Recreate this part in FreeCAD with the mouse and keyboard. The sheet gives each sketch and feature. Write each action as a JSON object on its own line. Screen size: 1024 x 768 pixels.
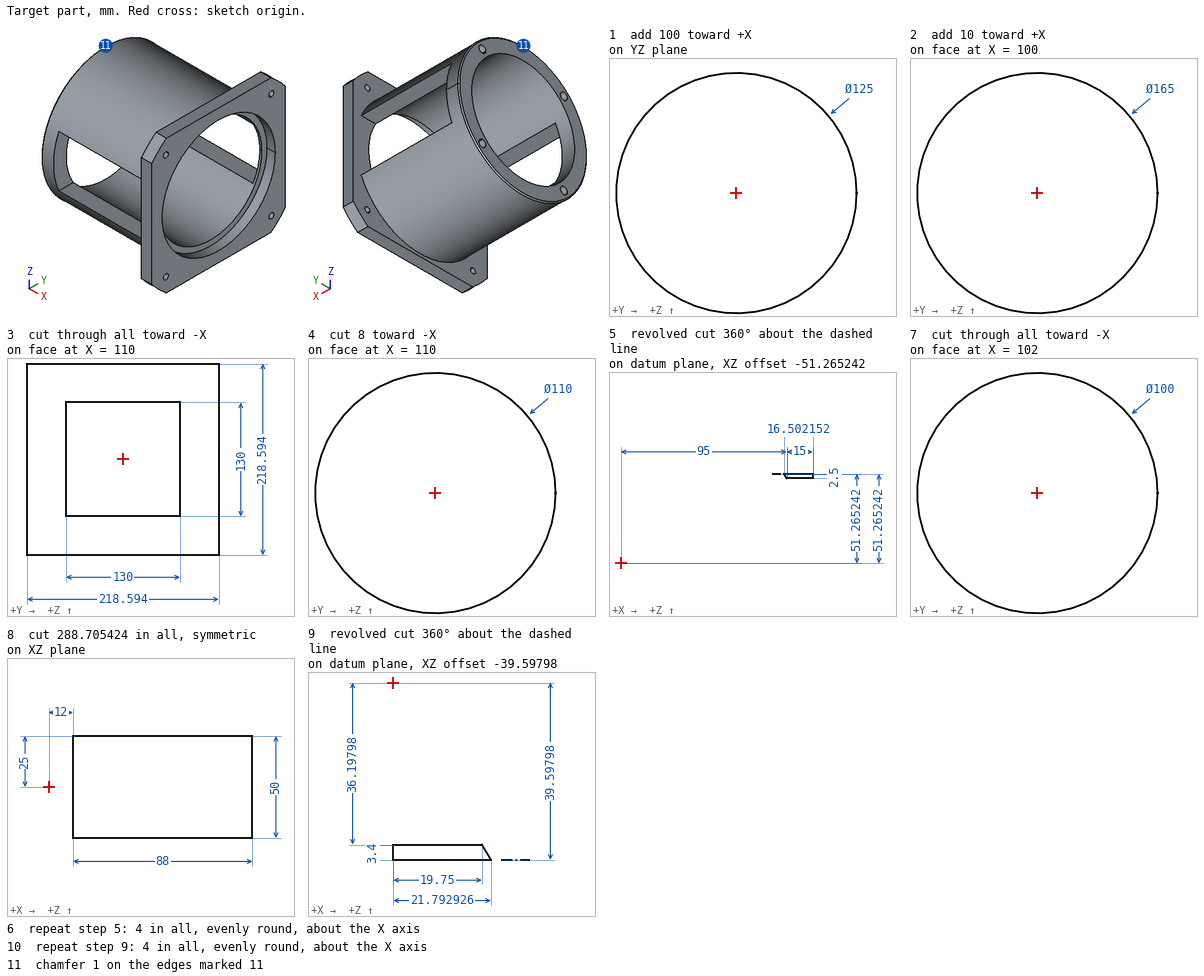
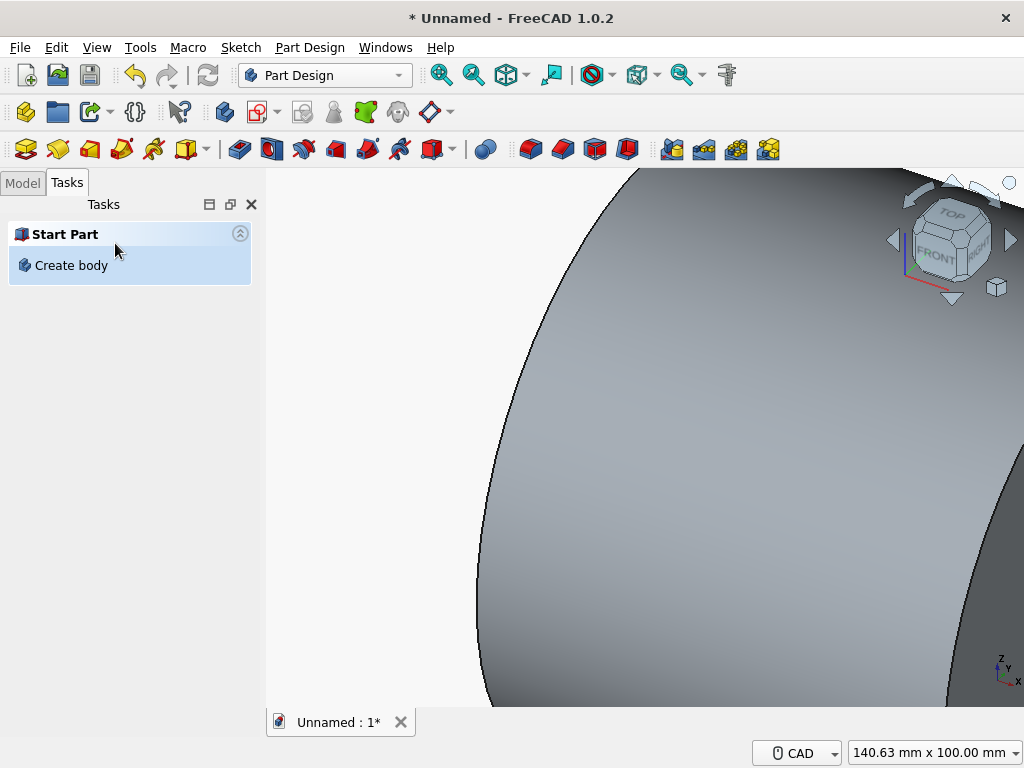
{"action": "left_click", "coordinate": [442, 76]}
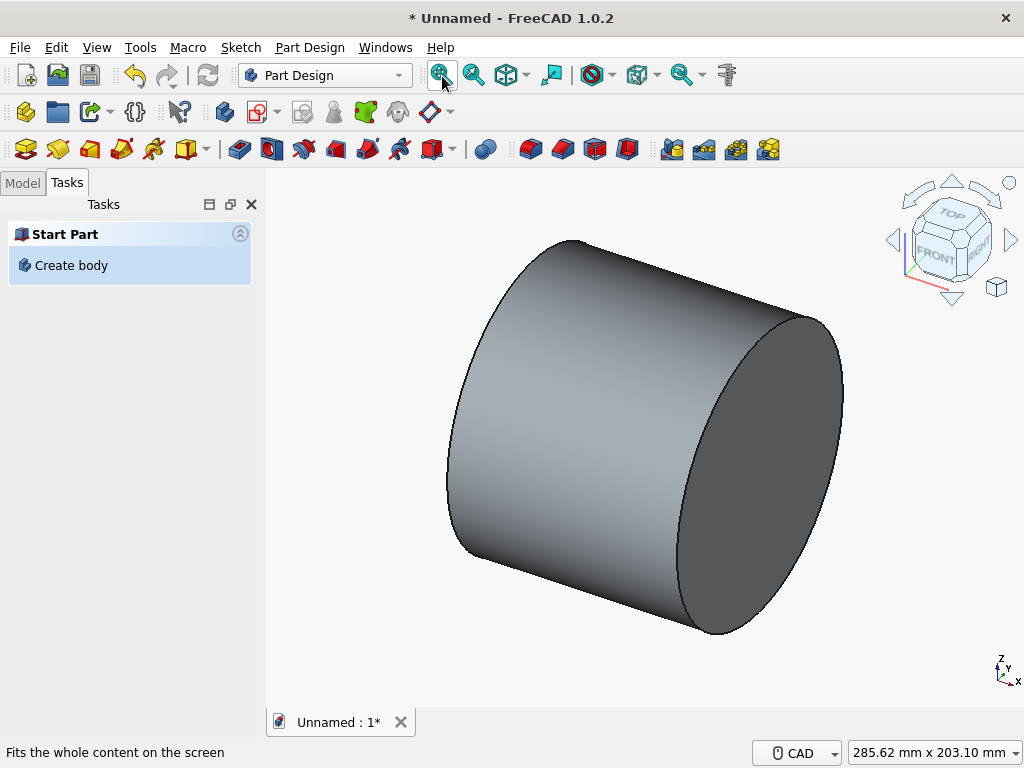
{"action": "left_click", "coordinate": [760, 475]}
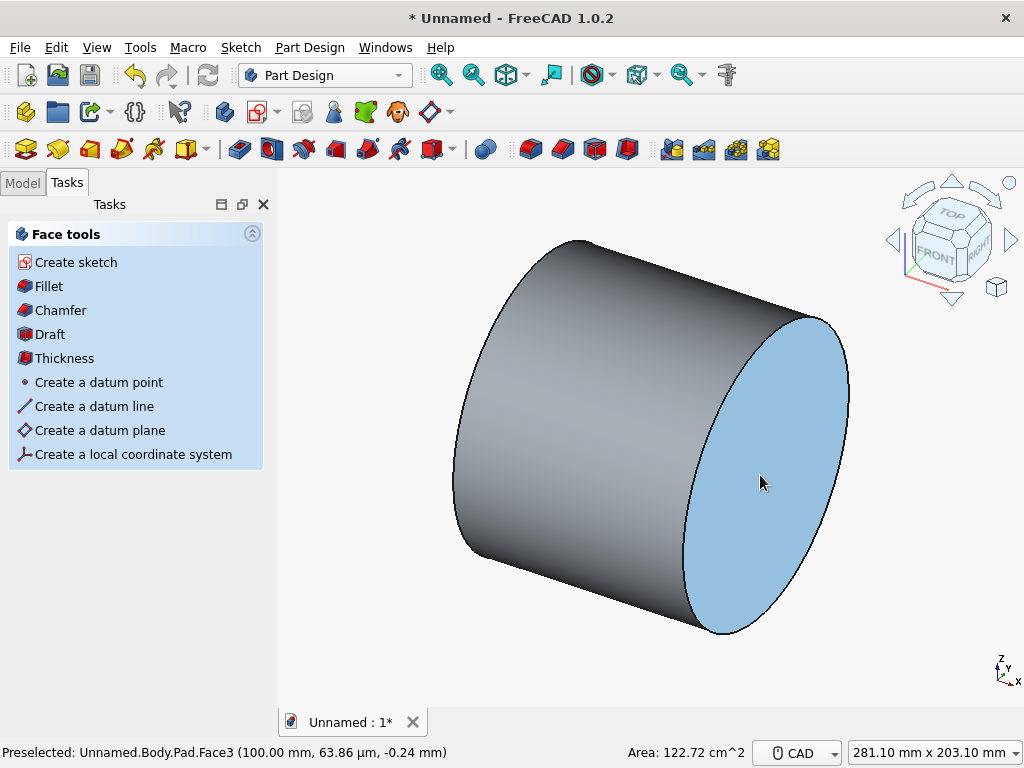
{"action": "left_click", "coordinate": [258, 112]}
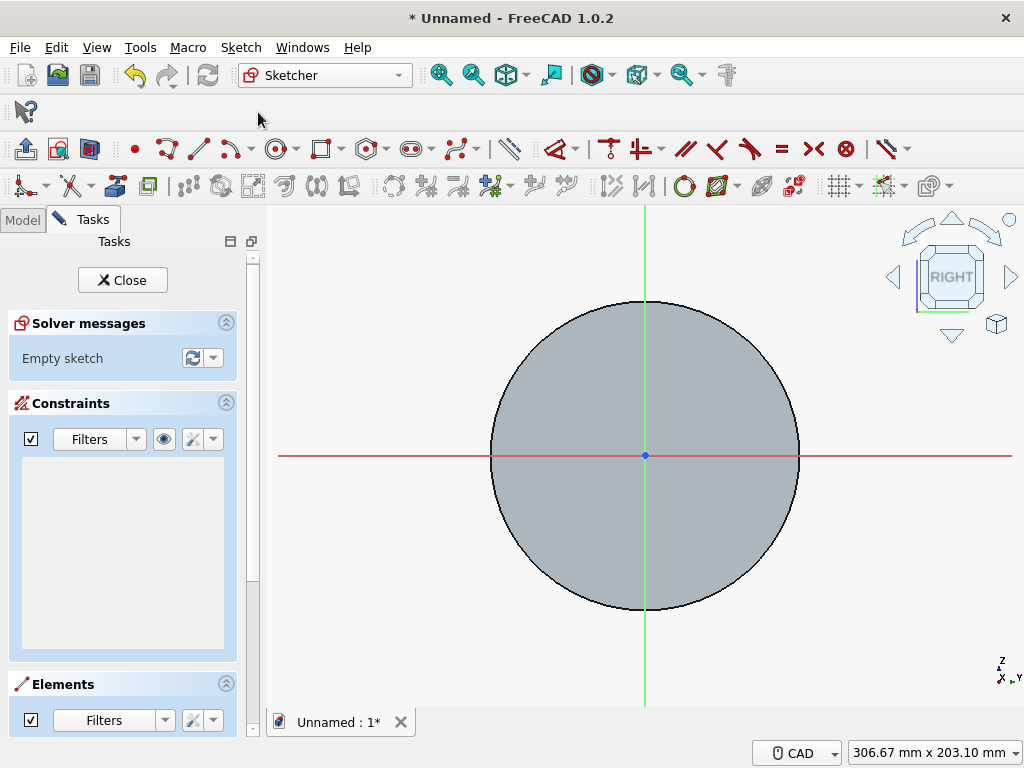
{"action": "scroll", "coordinate": [294, 456], "scroll_direction": "down", "scroll_amount": 1}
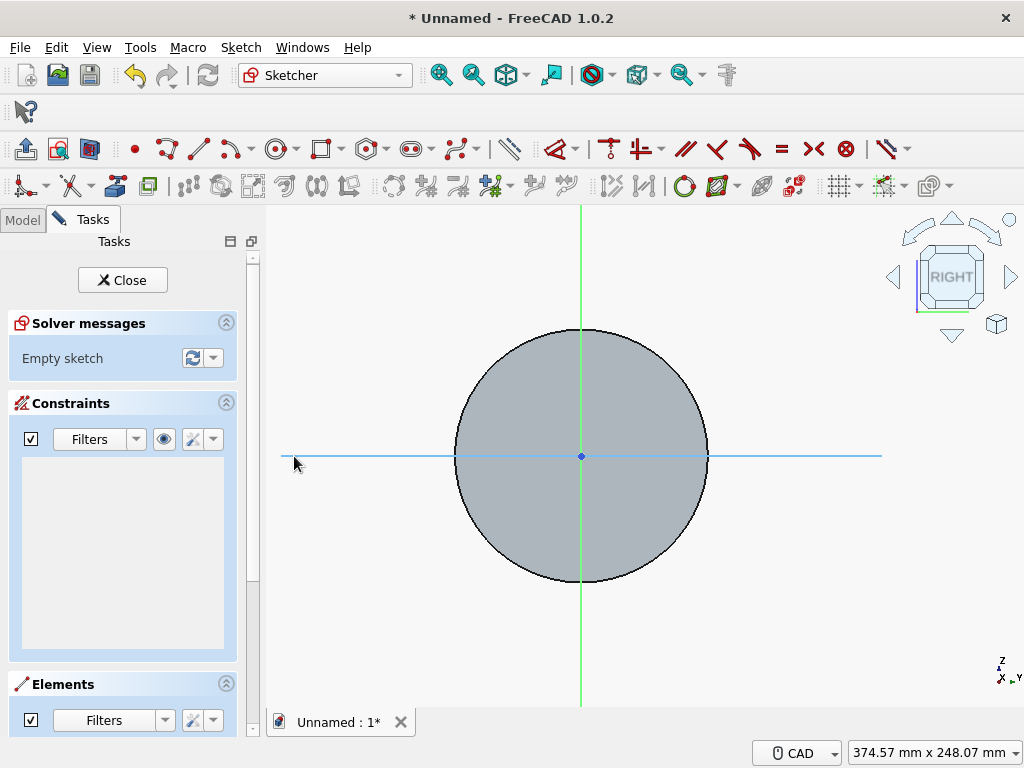
{"action": "left_click", "coordinate": [276, 150]}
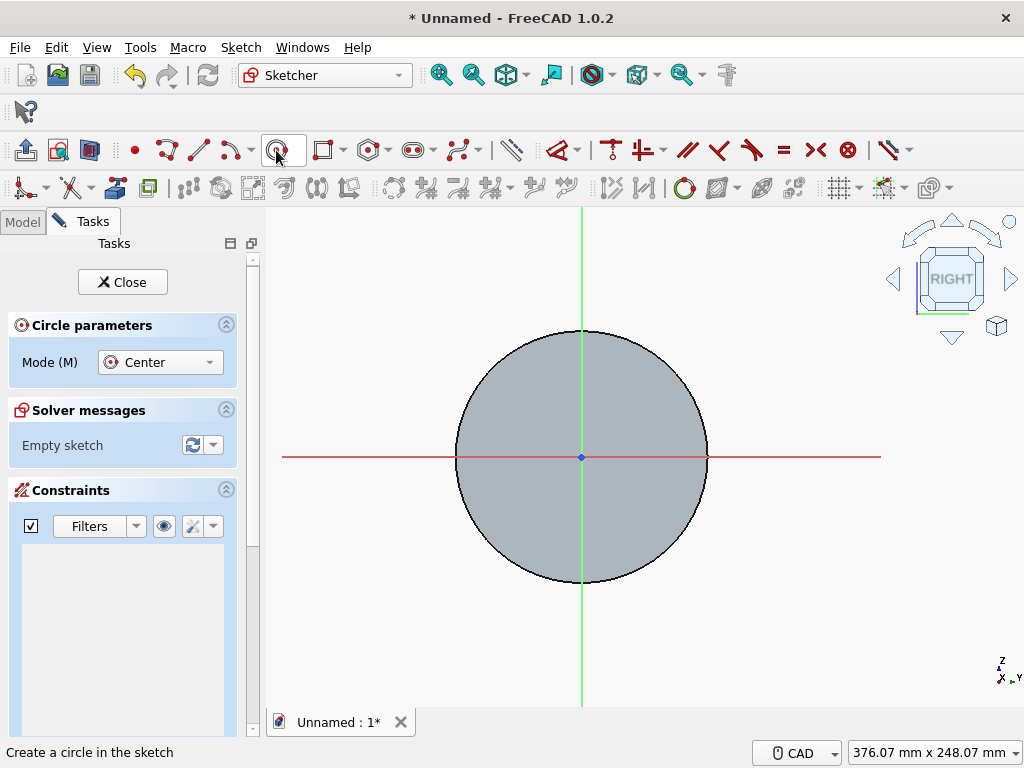
{"action": "left_click", "coordinate": [582, 457]}
{"action": "mouse_move", "coordinate": [699, 340]}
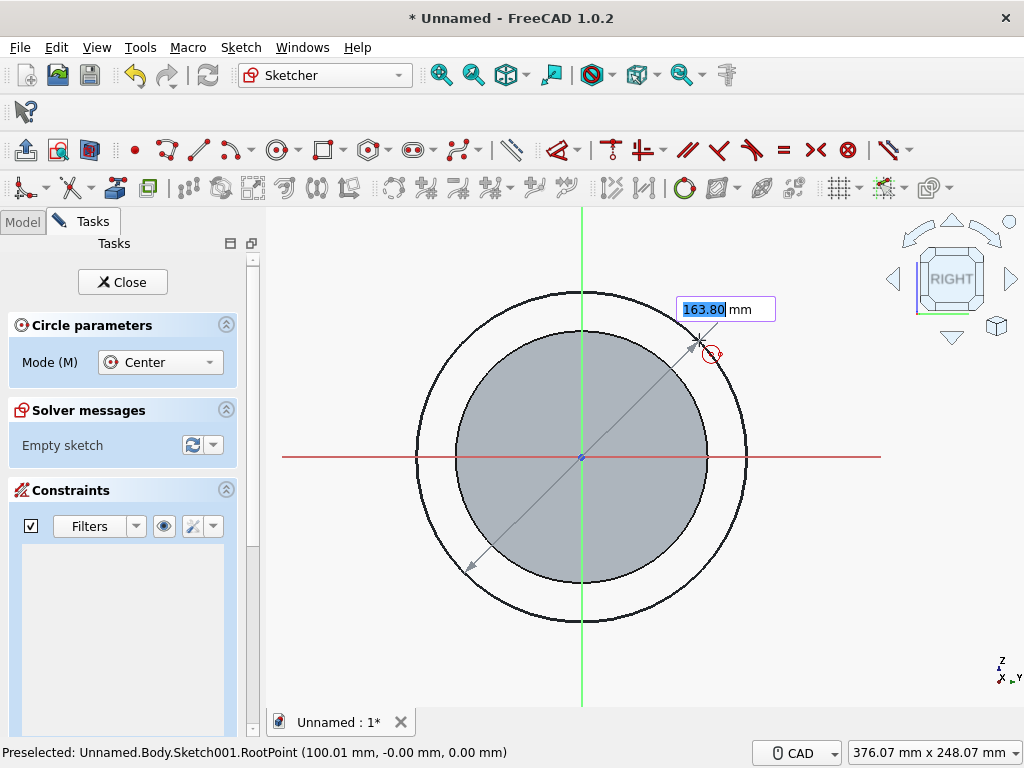
{"action": "type", "text": "165"}
{"action": "key", "text": "Return"}
{"action": "key", "text": "Escape"}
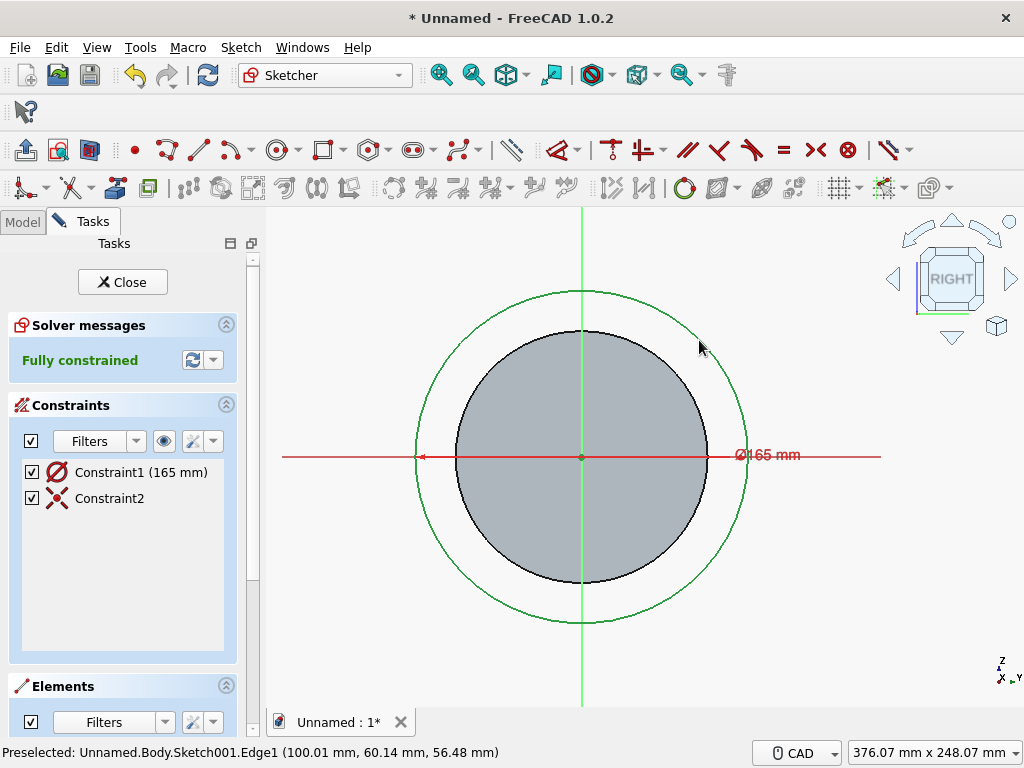
{"action": "left_click", "coordinate": [123, 282]}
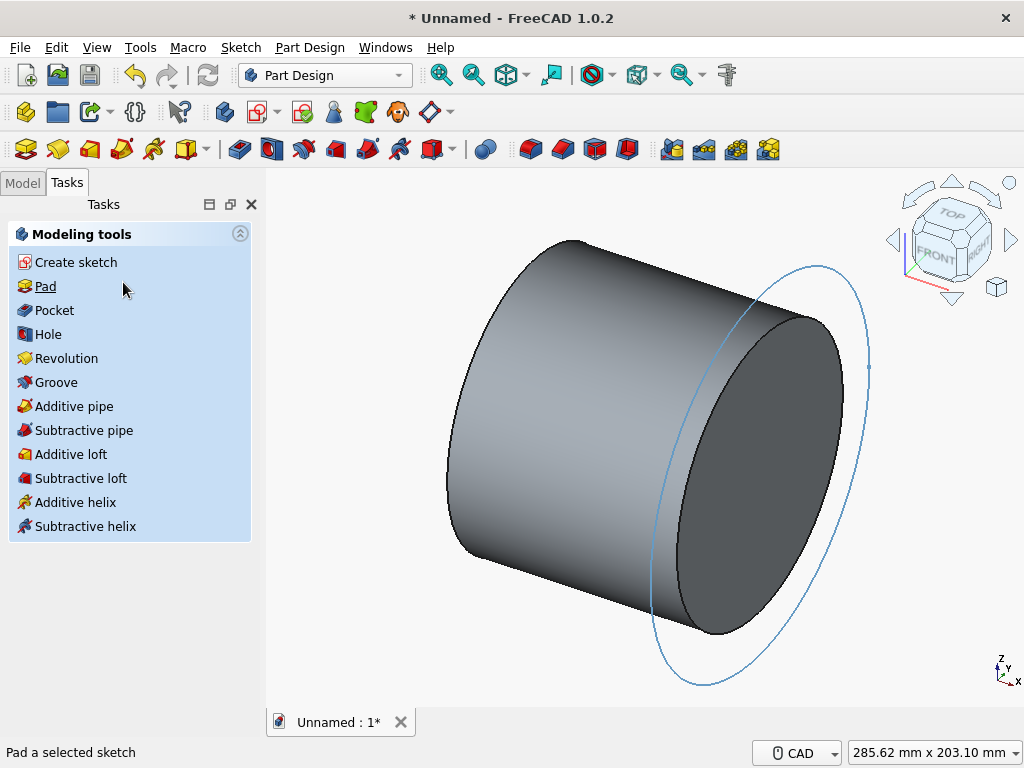
{"action": "left_click", "coordinate": [26, 150]}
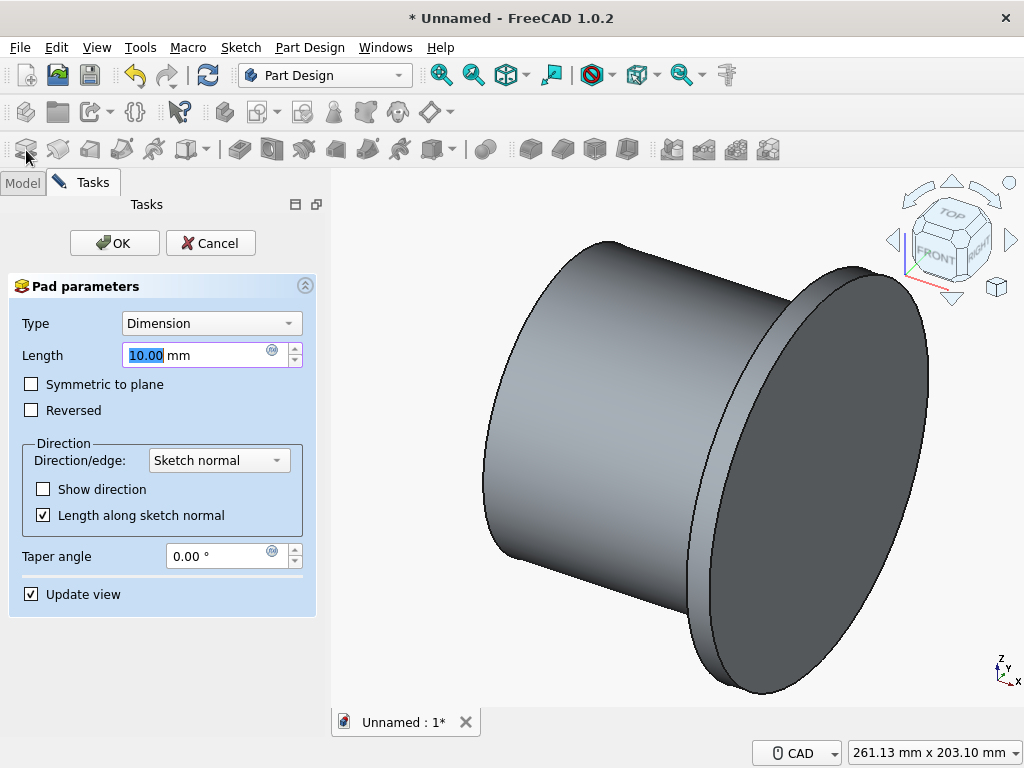
{"action": "type", "text": "10"}
{"action": "key", "text": "Tab"}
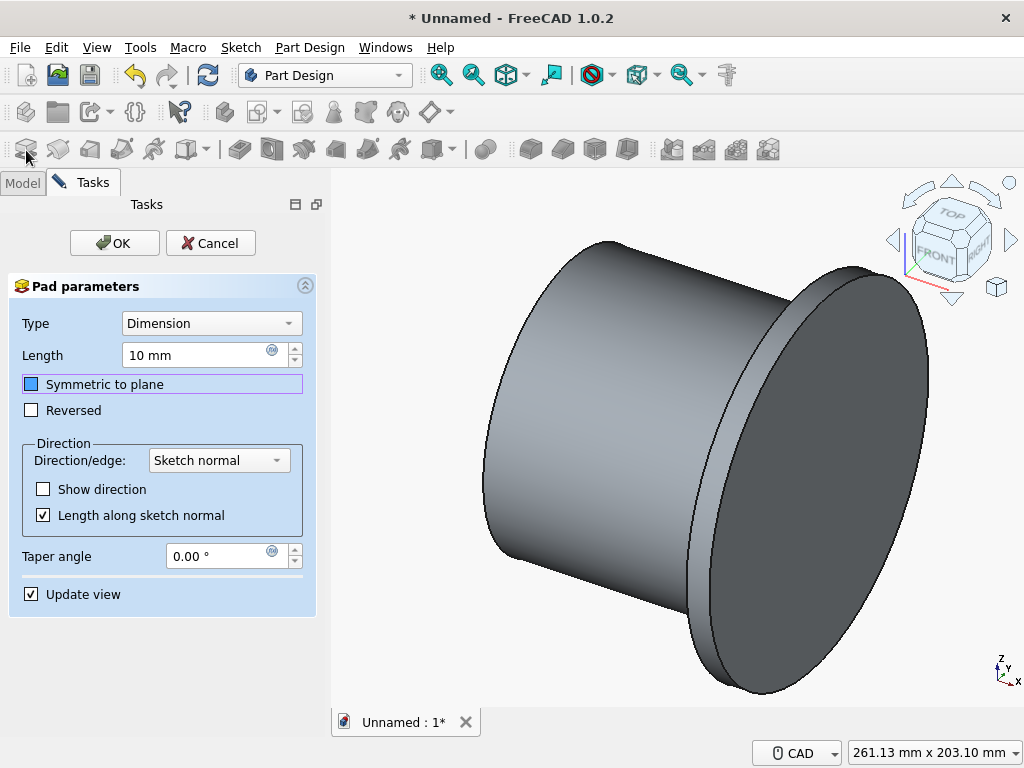
{"action": "left_click", "coordinate": [115, 243]}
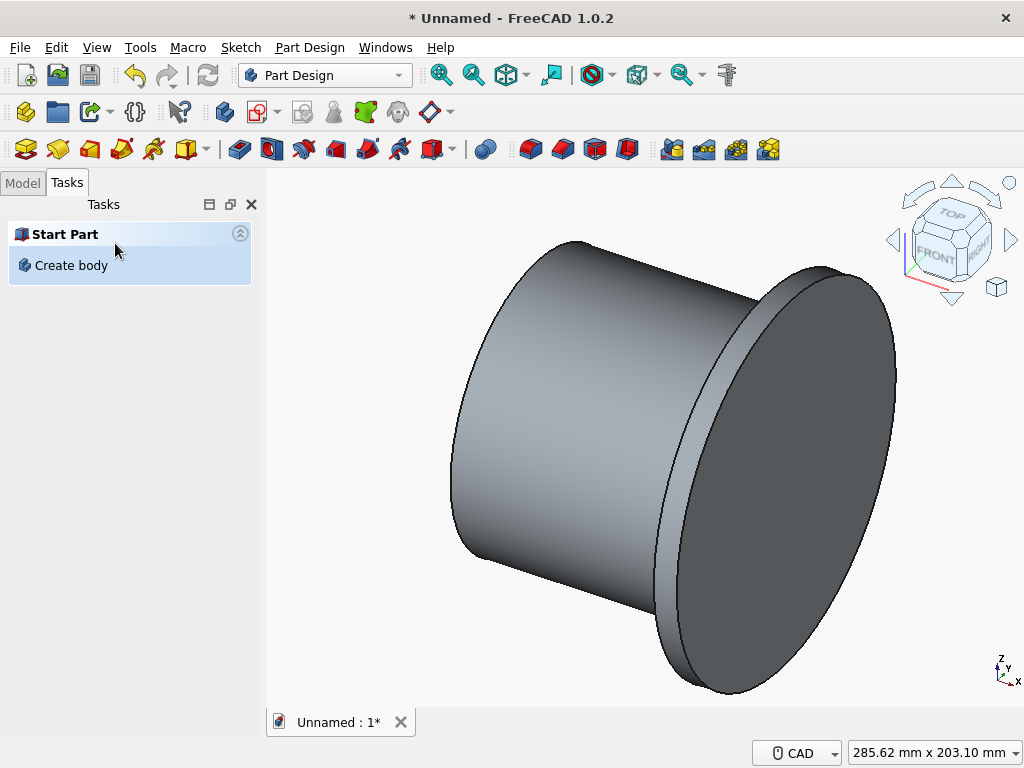
{"action": "left_click", "coordinate": [442, 76]}